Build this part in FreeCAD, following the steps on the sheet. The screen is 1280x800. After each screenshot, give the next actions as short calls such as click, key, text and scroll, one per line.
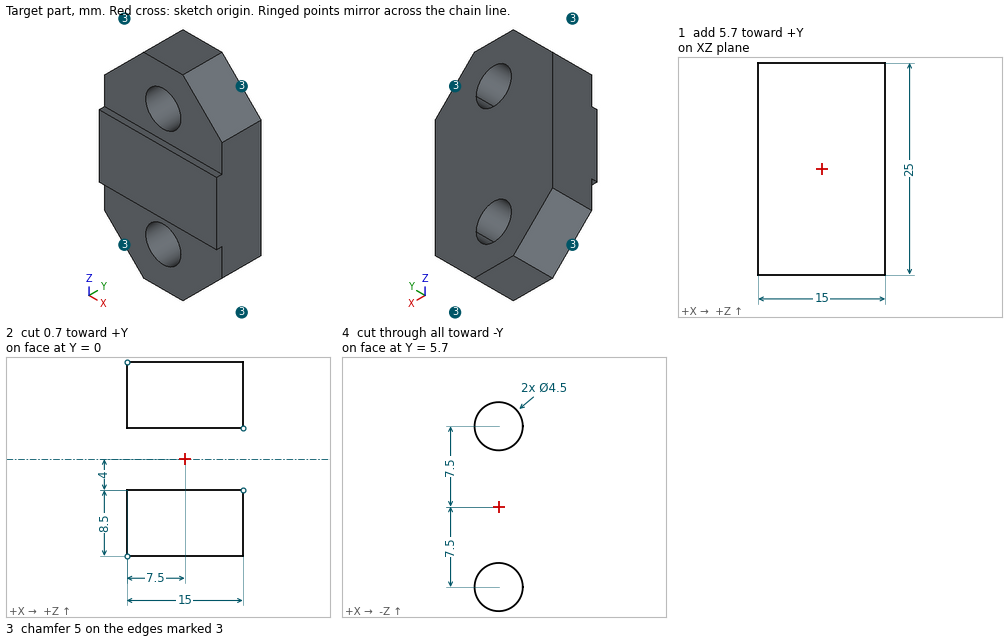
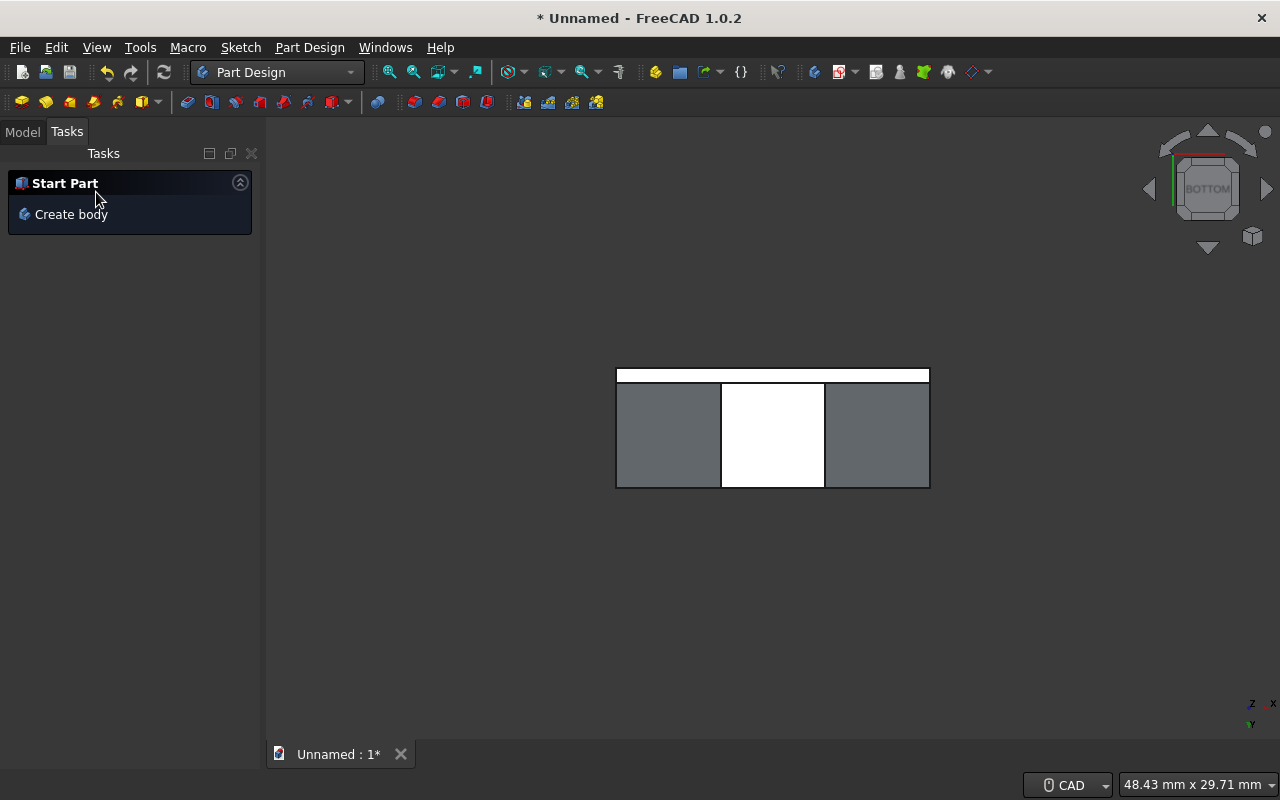
key(v)
key(f)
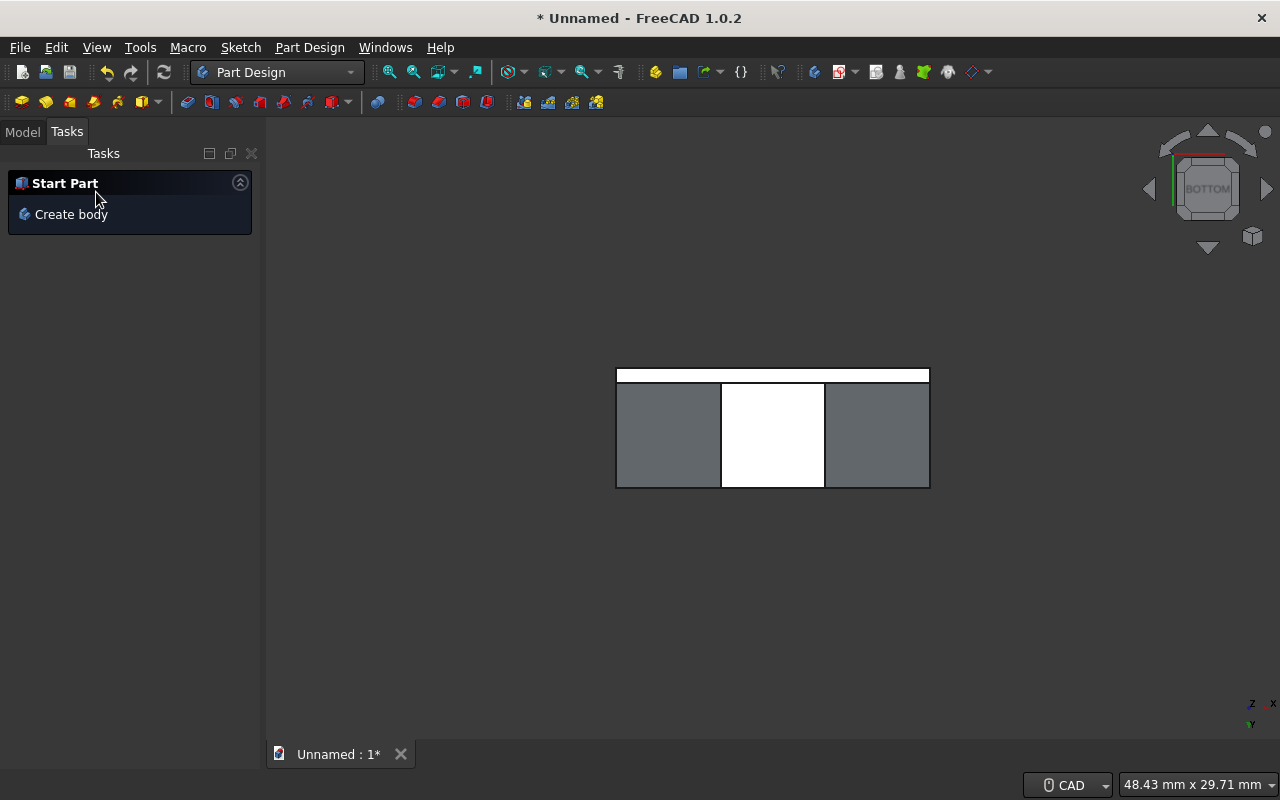
key(4)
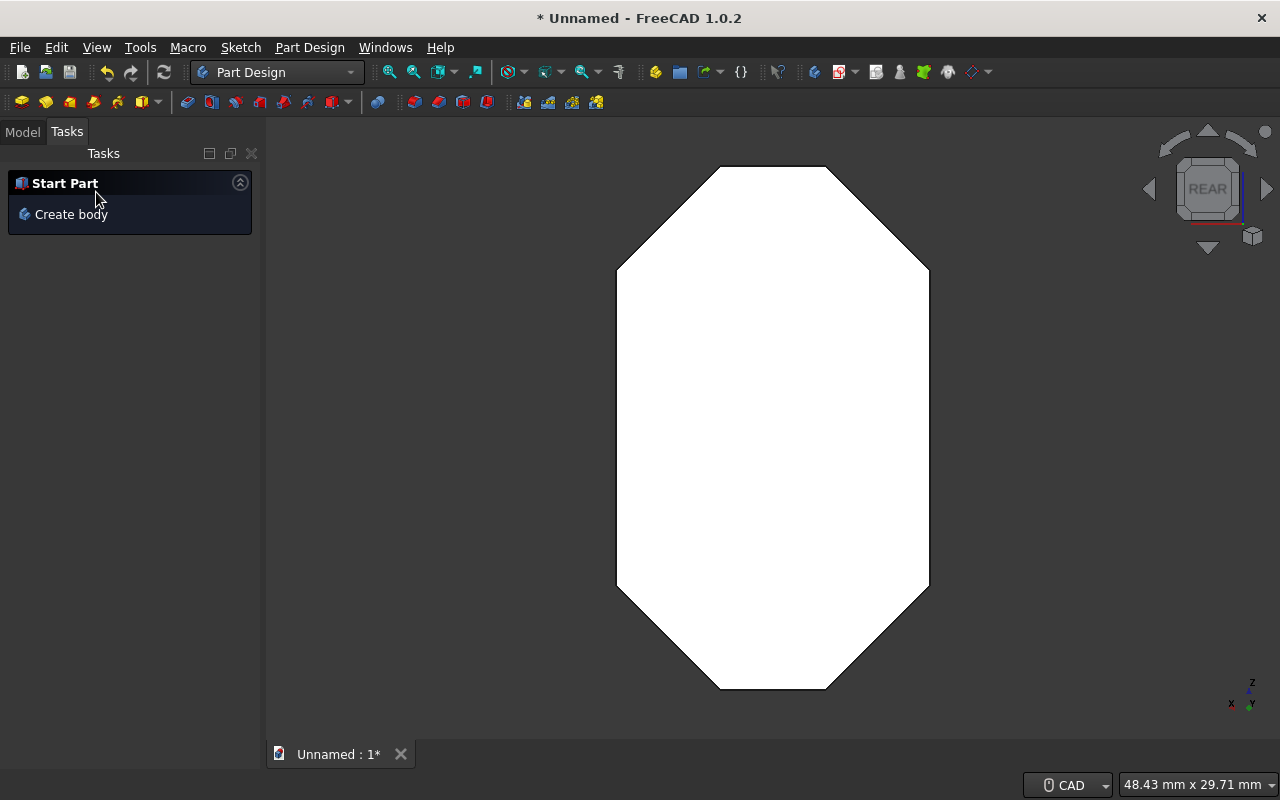
click(773, 352)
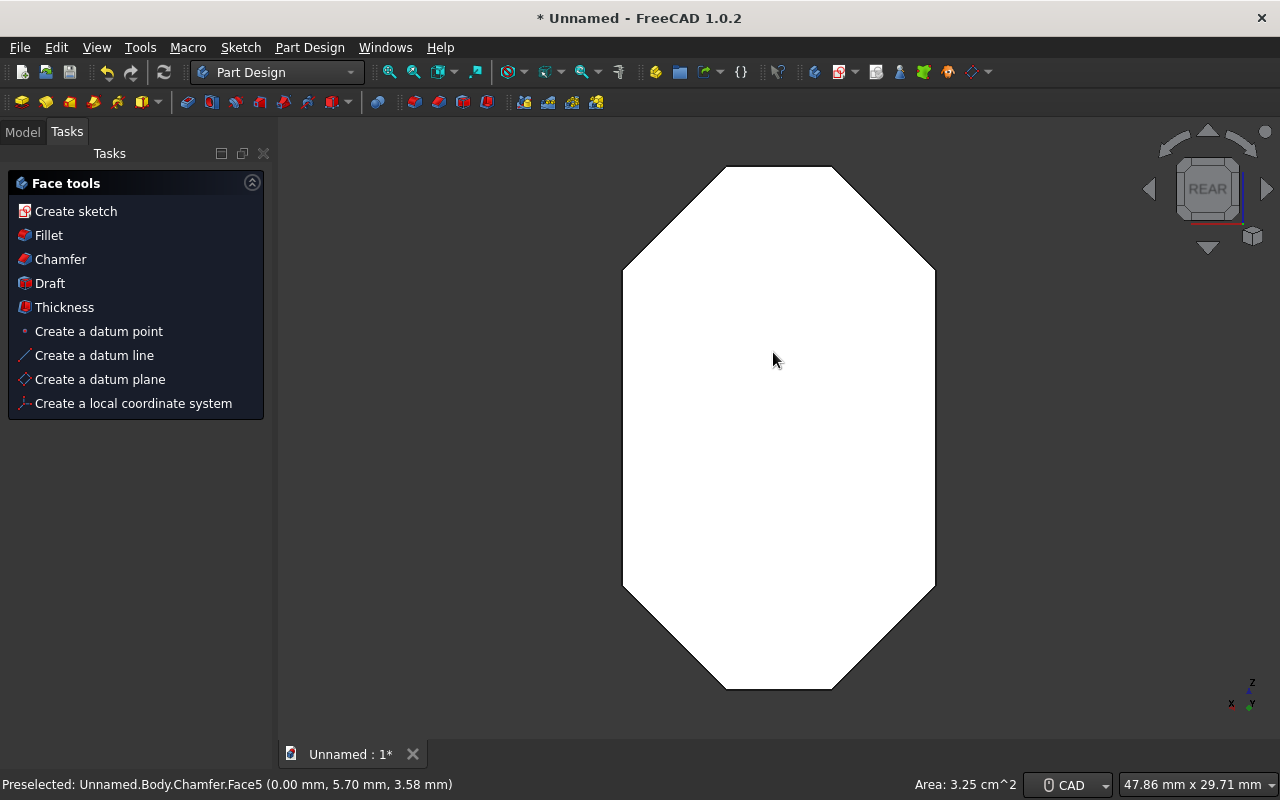
click(840, 72)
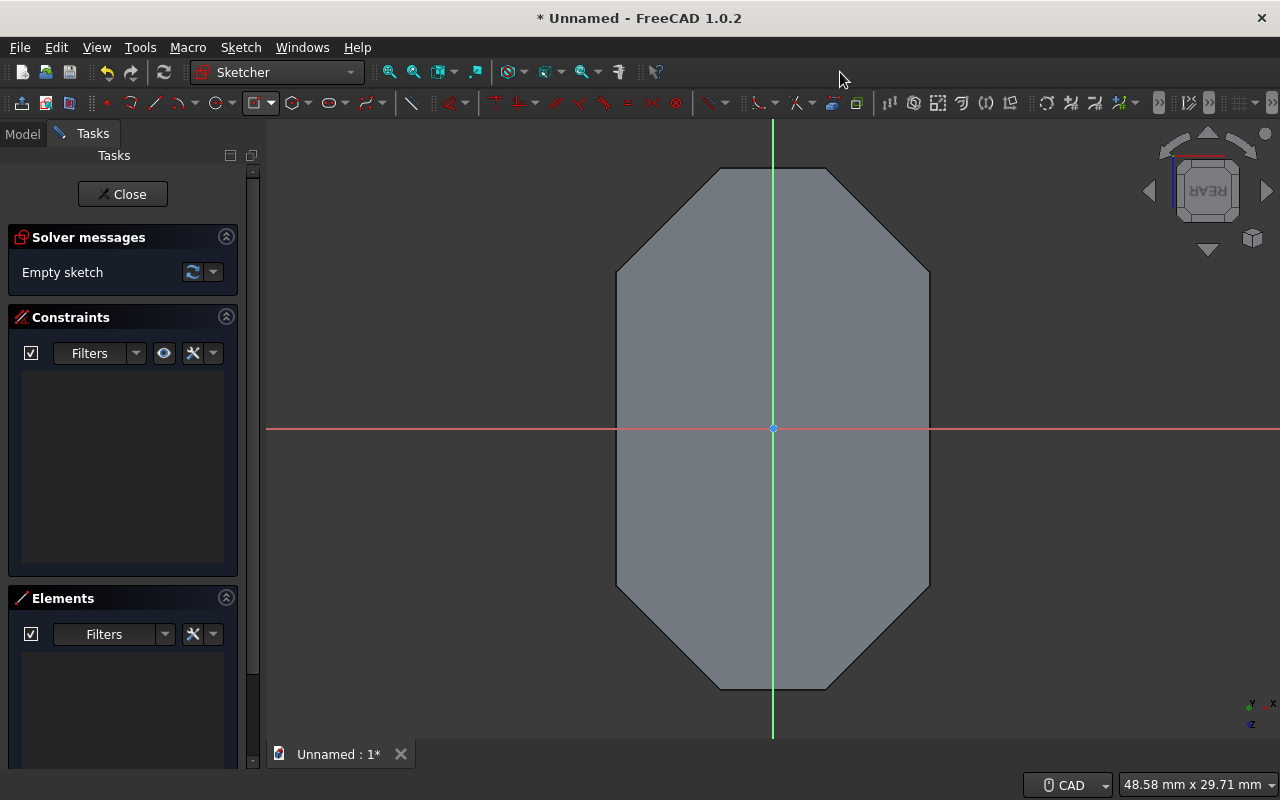
key(g)
key(c)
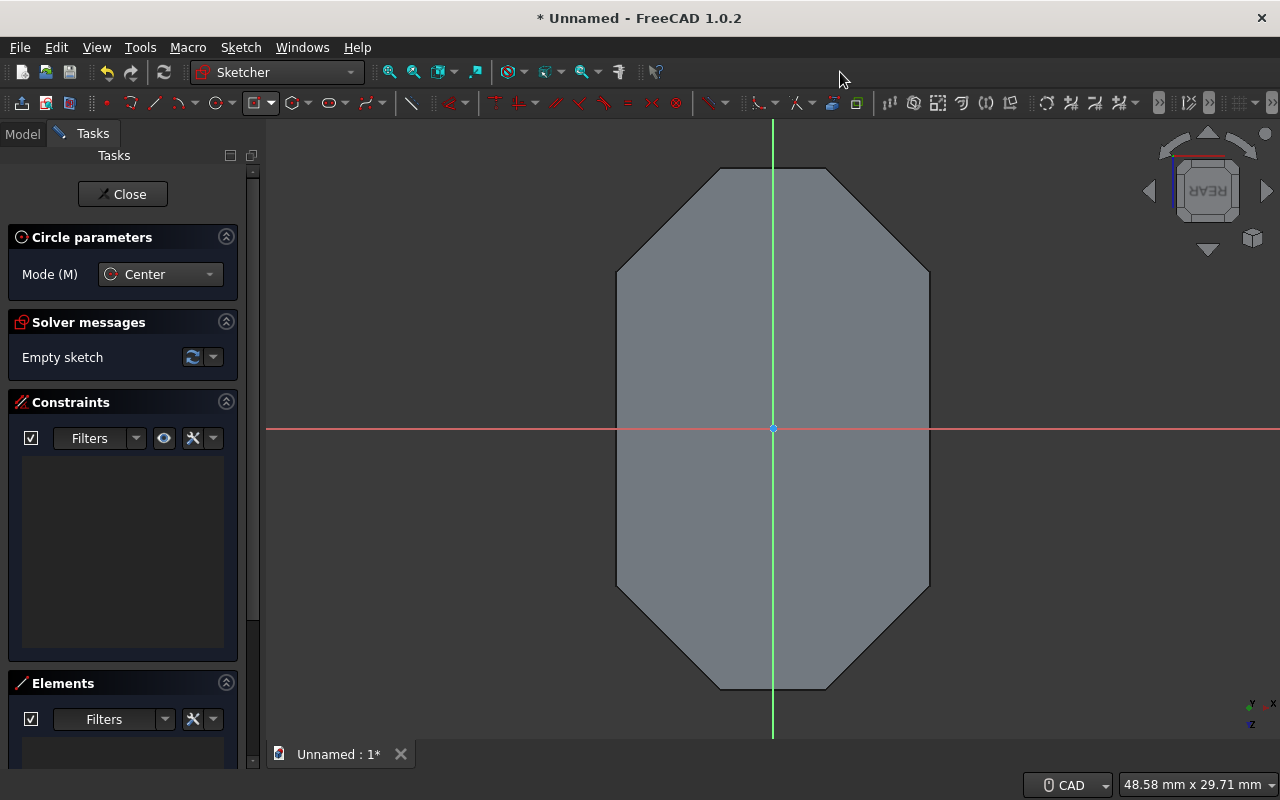
click(773, 272)
click(806, 239)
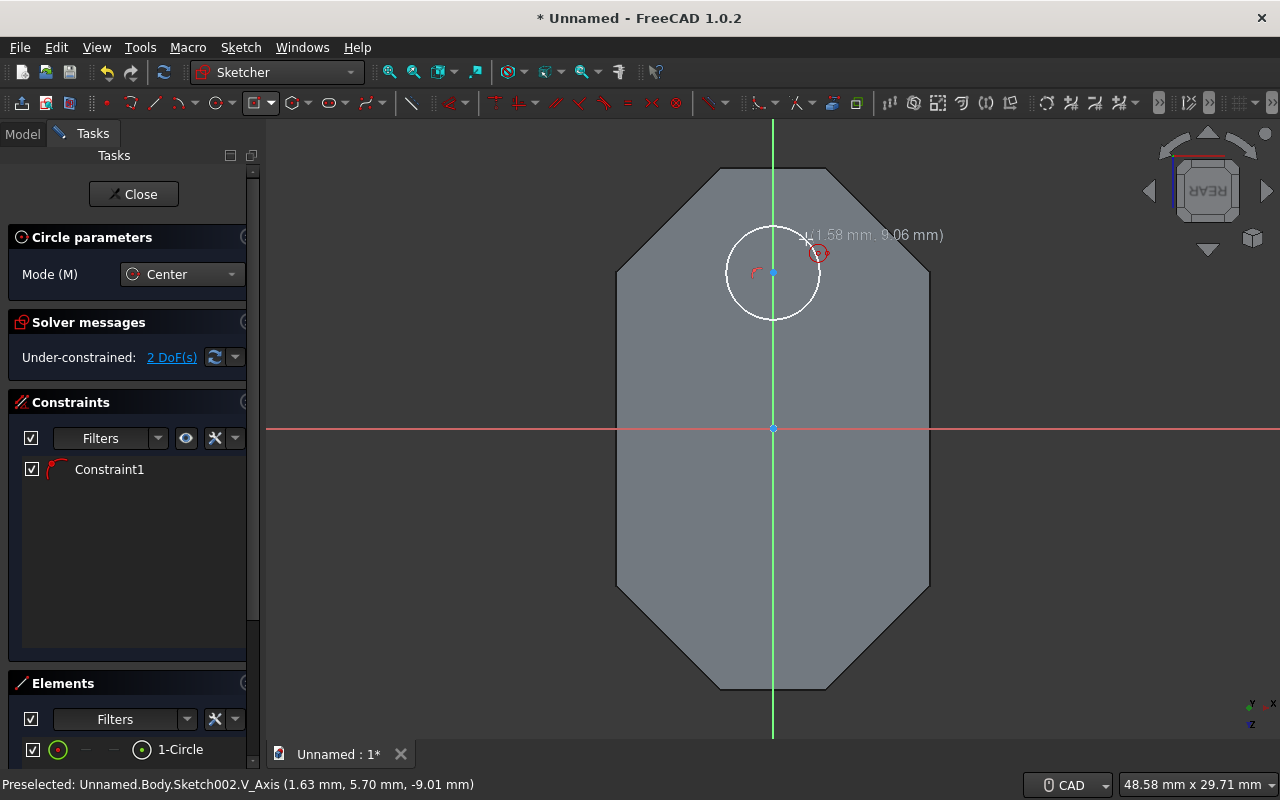
click(773, 586)
click(806, 552)
key(Escape)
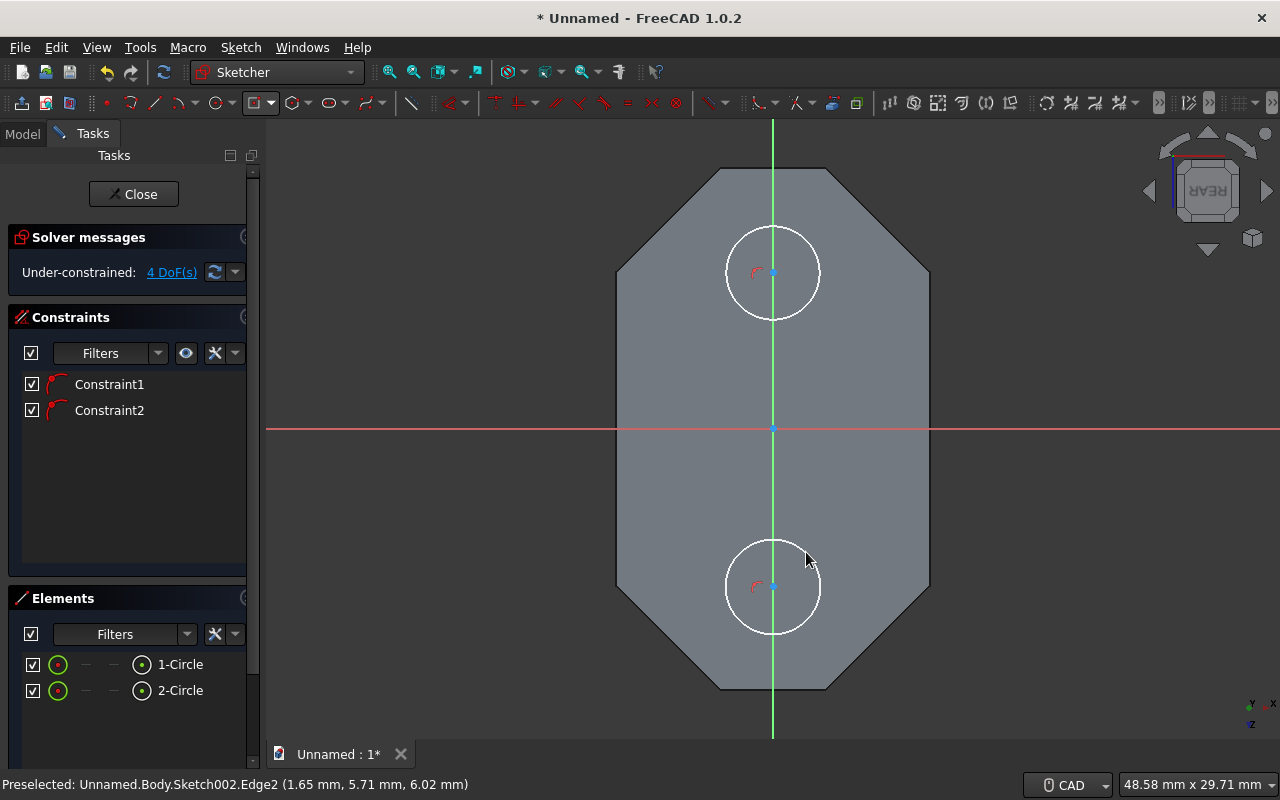
click(806, 240)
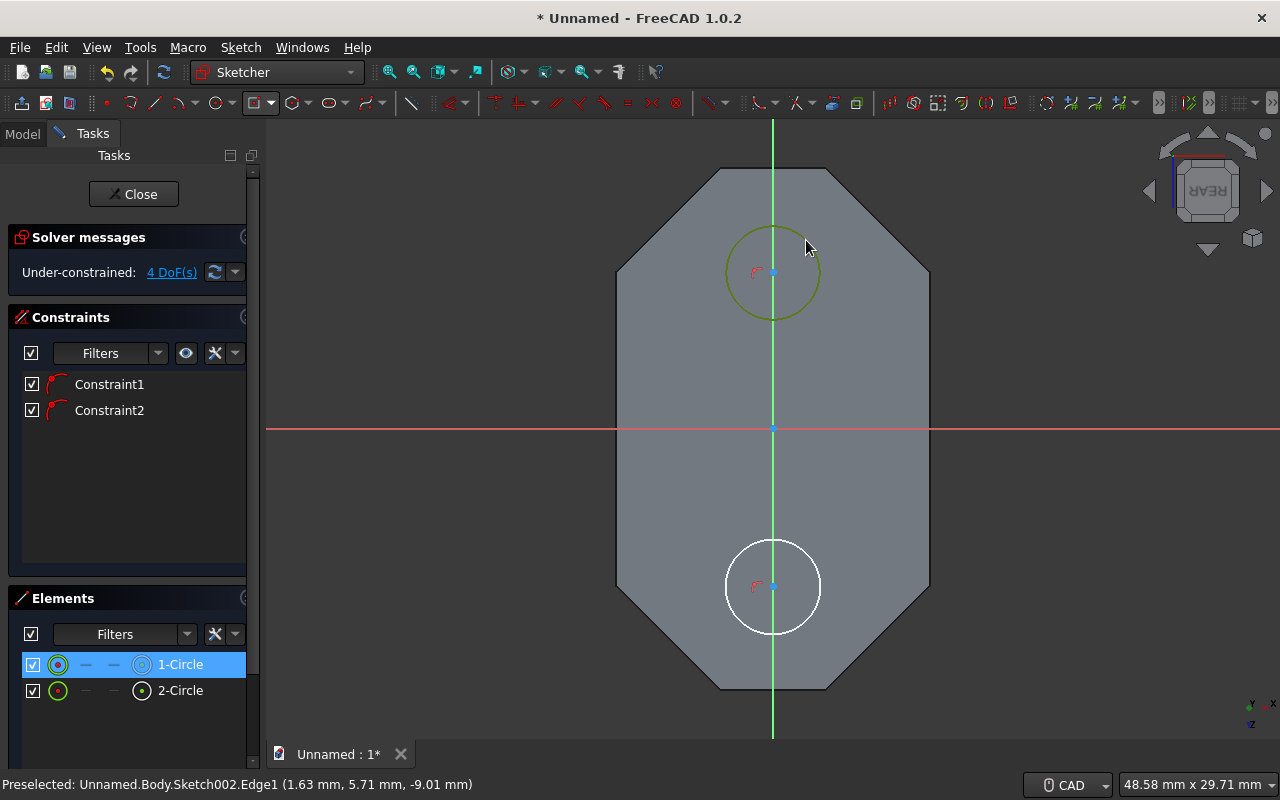
click(806, 553)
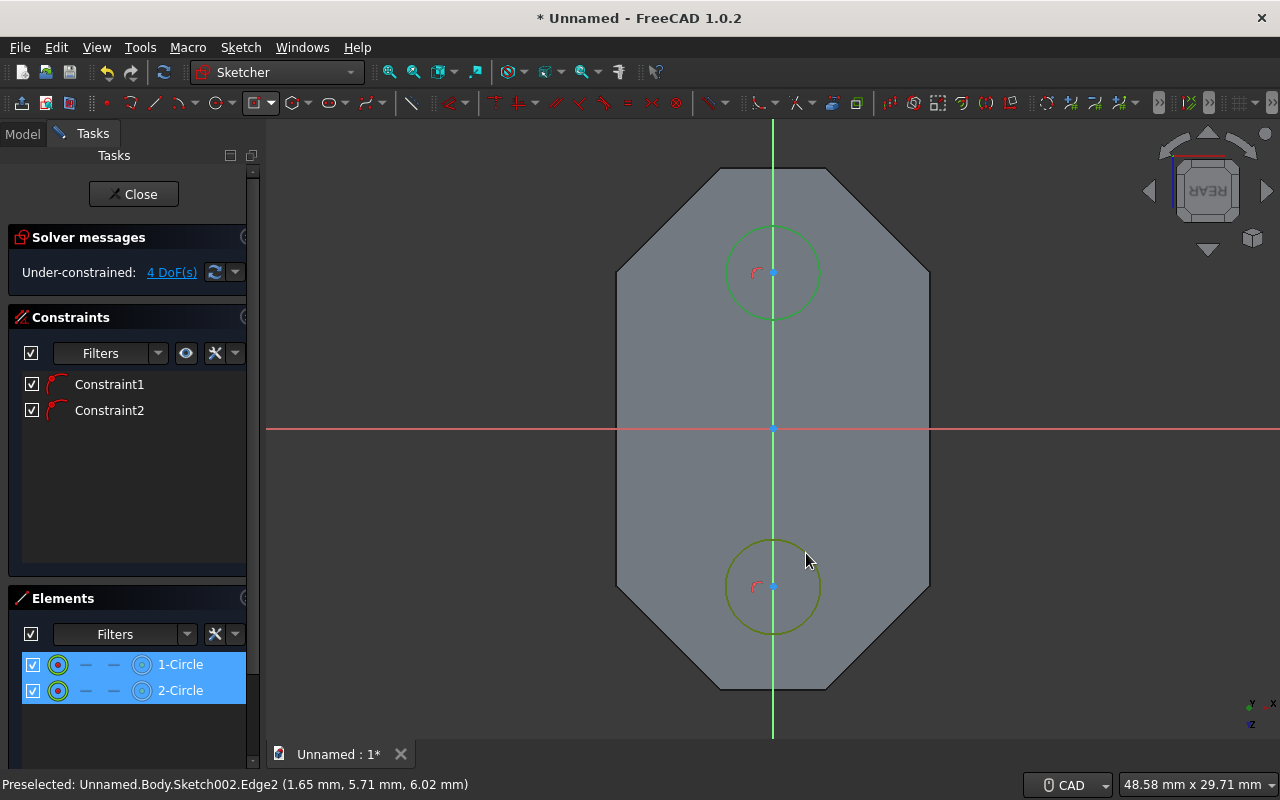
click(628, 104)